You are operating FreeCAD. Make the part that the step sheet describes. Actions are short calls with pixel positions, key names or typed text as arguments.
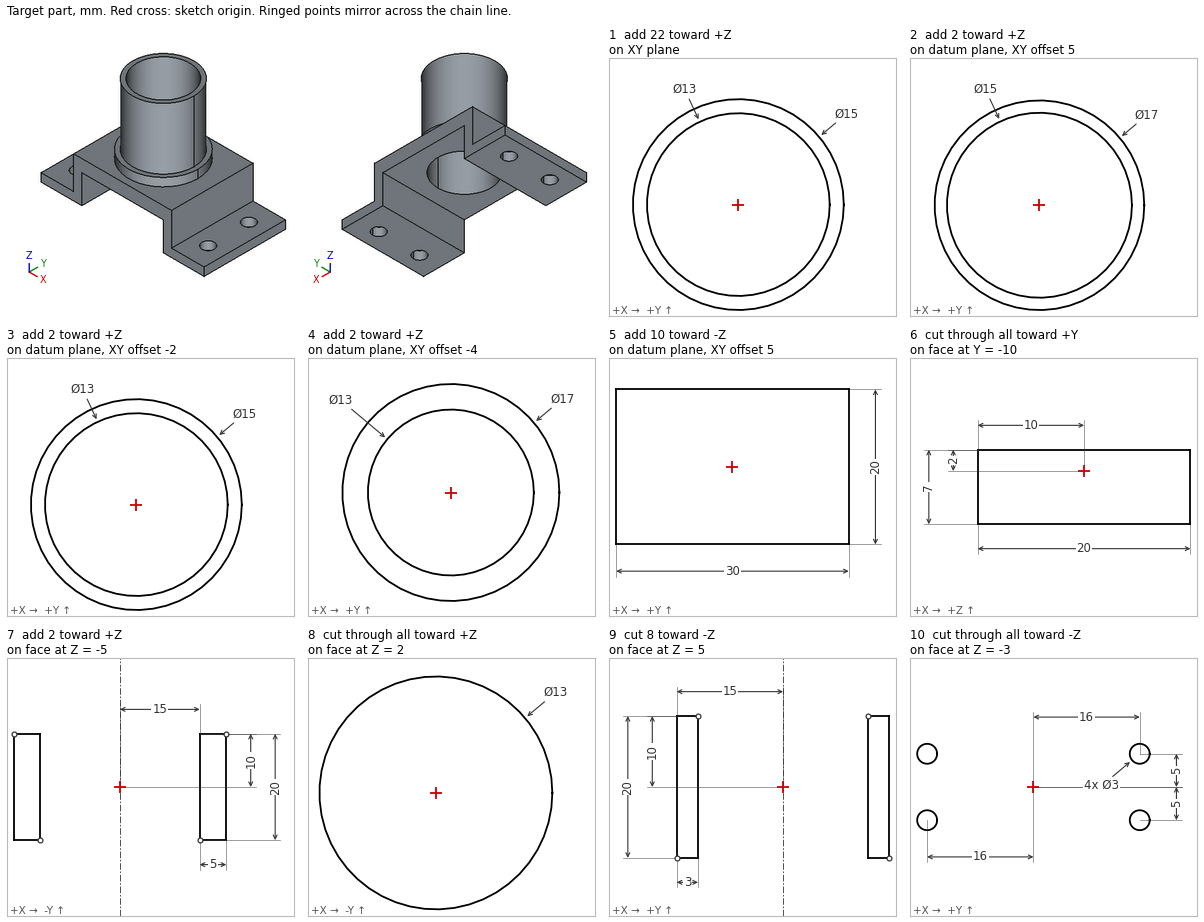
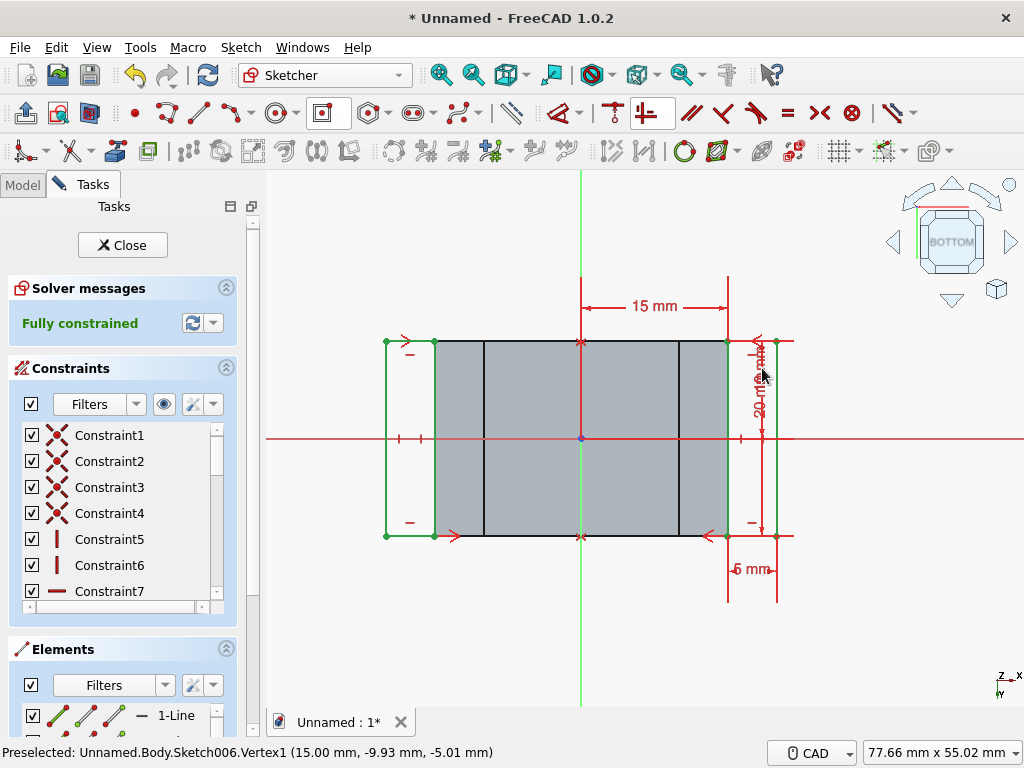
click(123, 245)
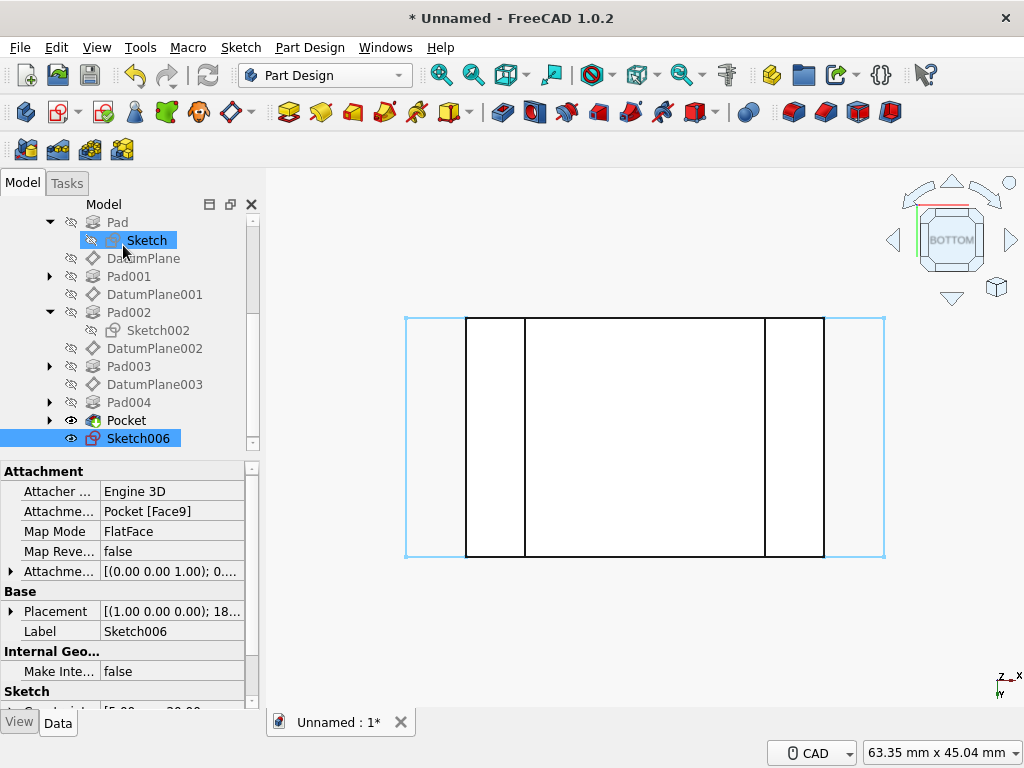
click(290, 112)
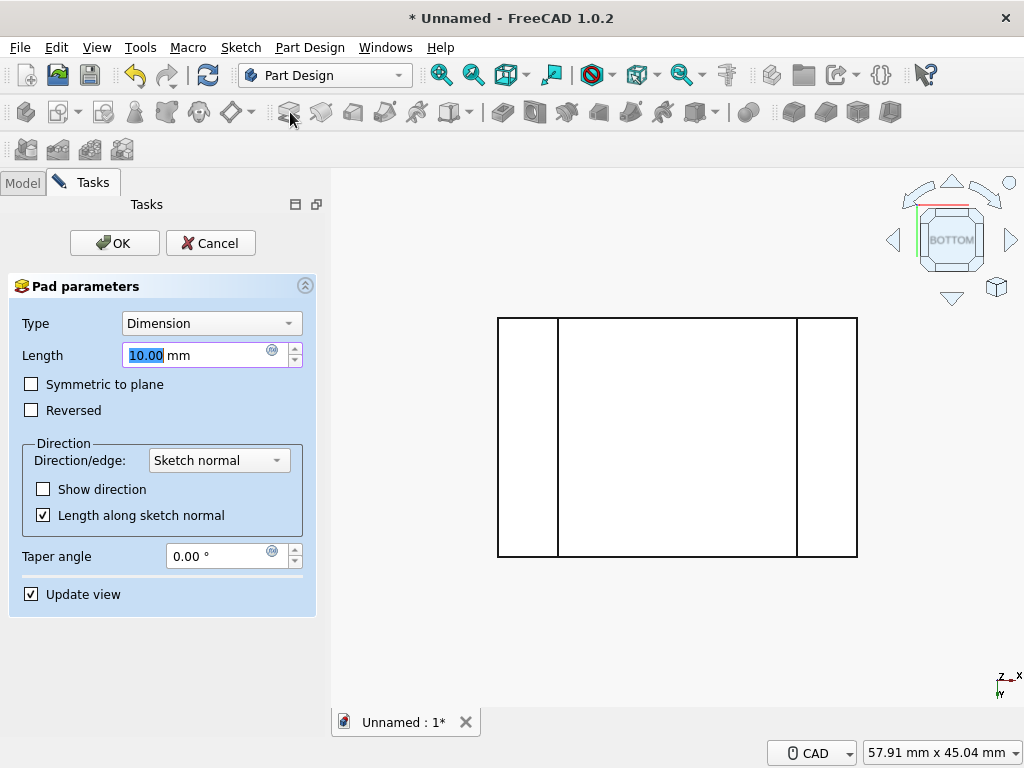
text(2)
key(Tab)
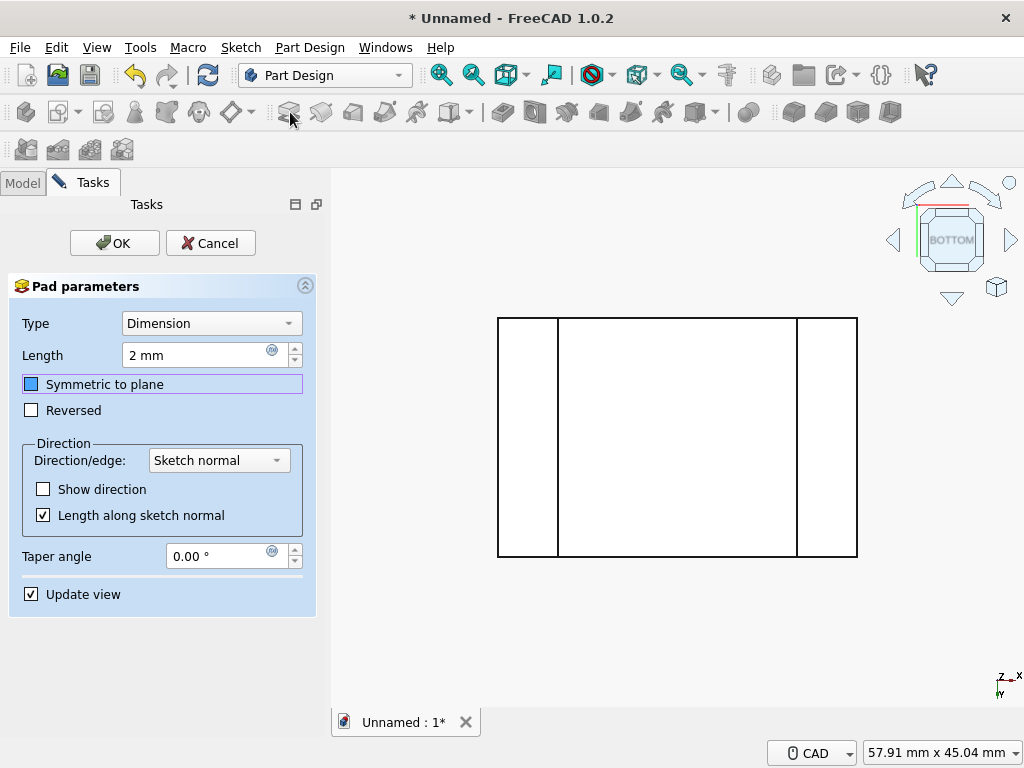
click(30, 410)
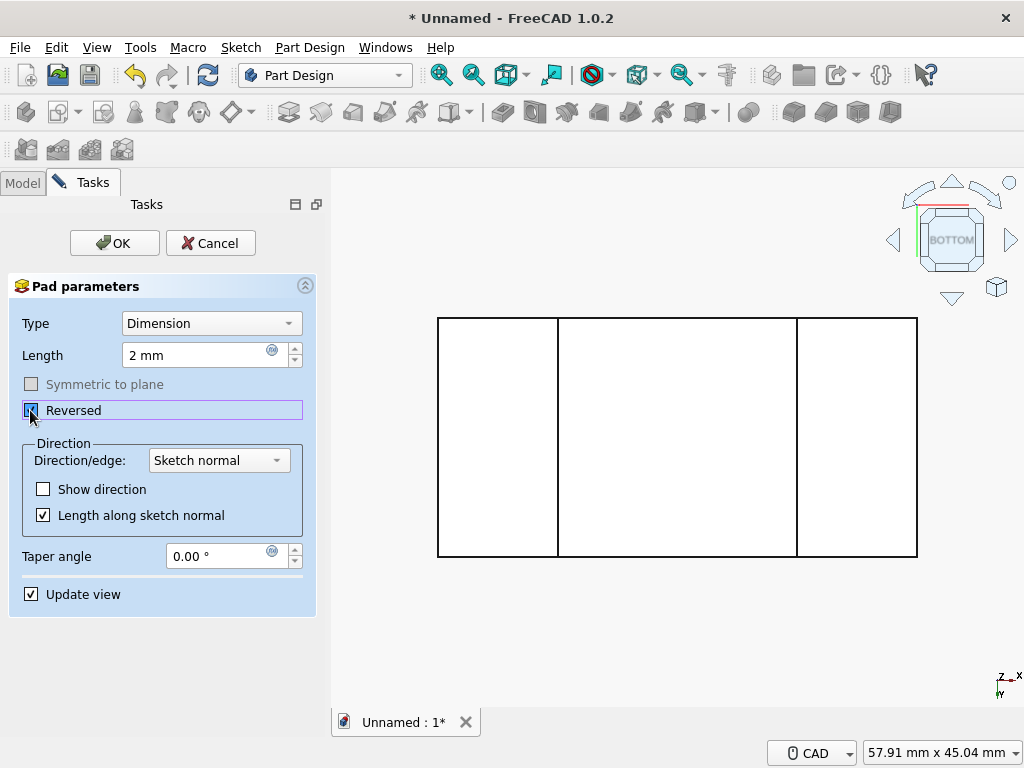
click(115, 243)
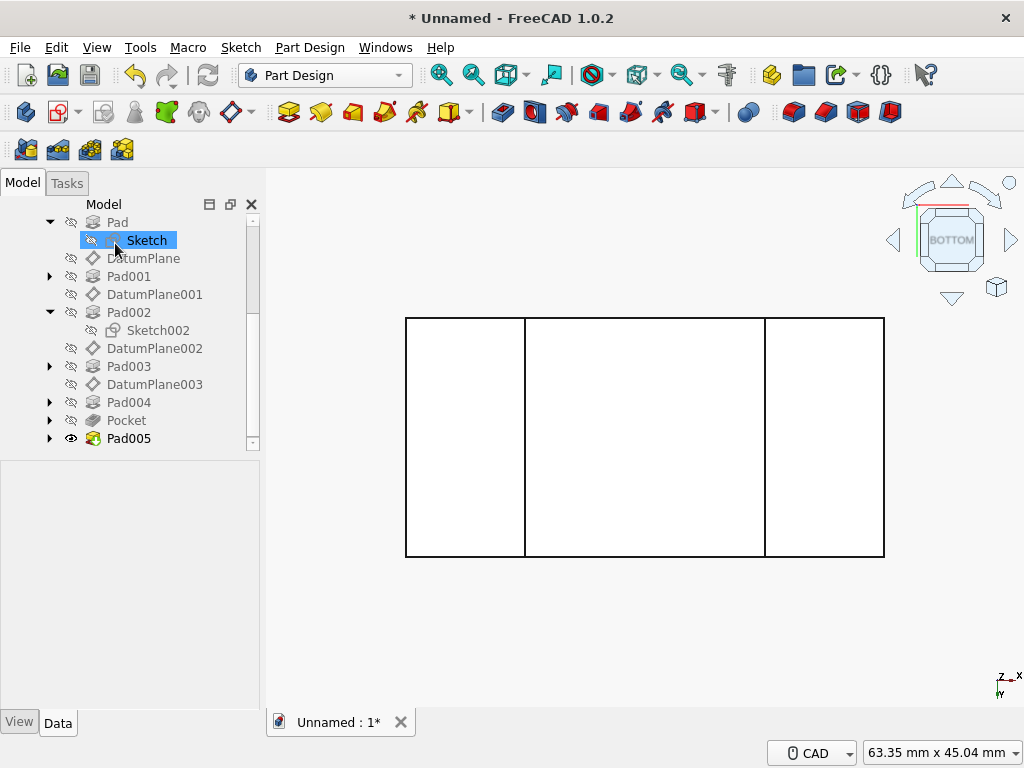
click(645, 437)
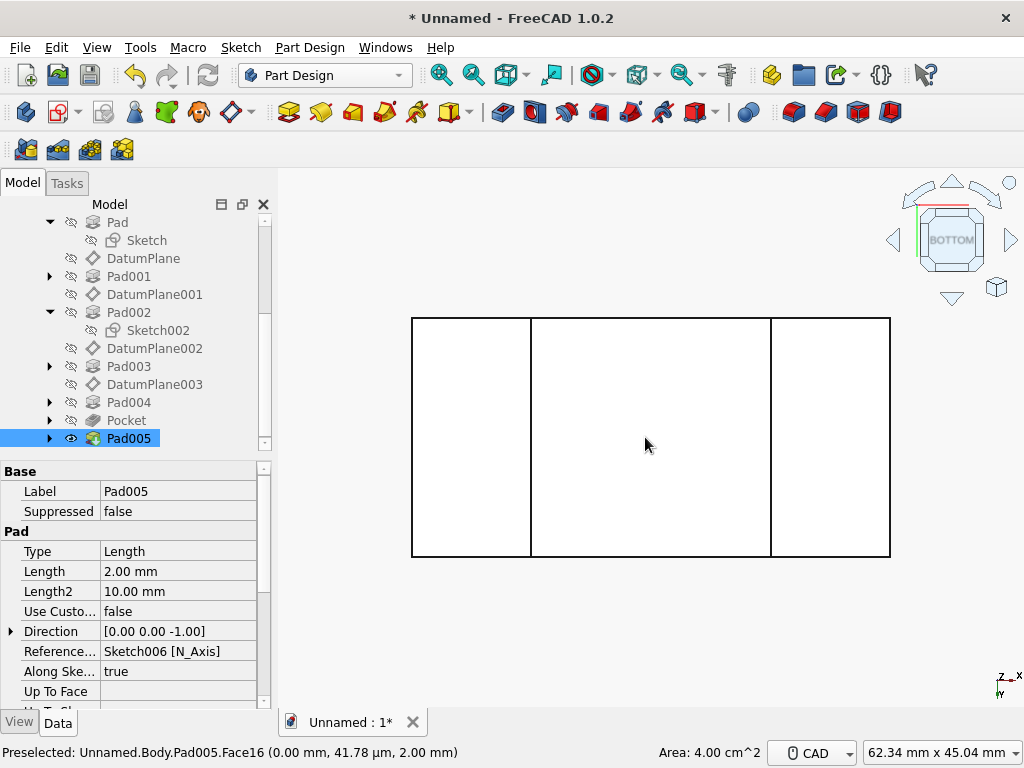
click(58, 112)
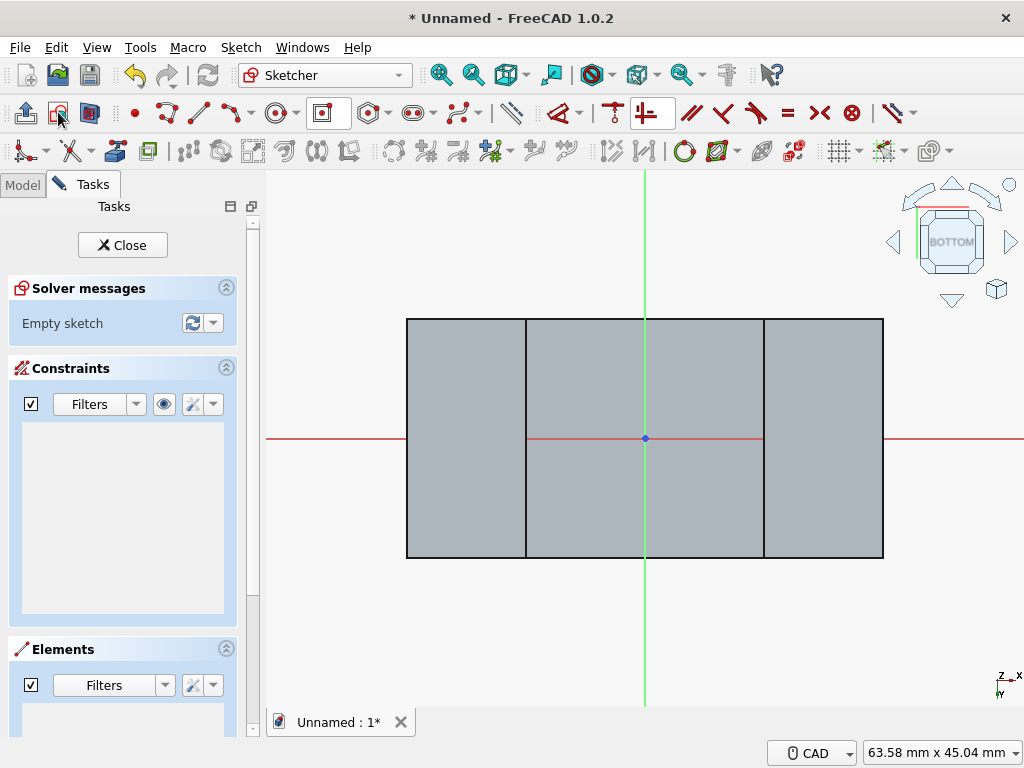
click(90, 114)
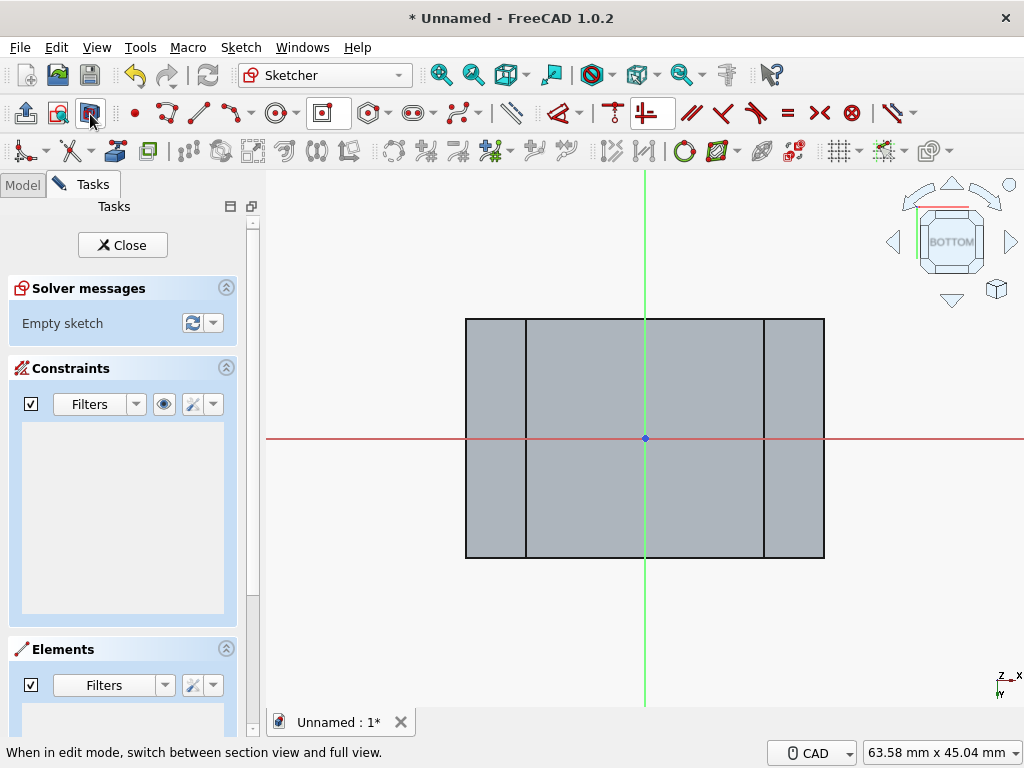
scroll(701, 439, up, 4)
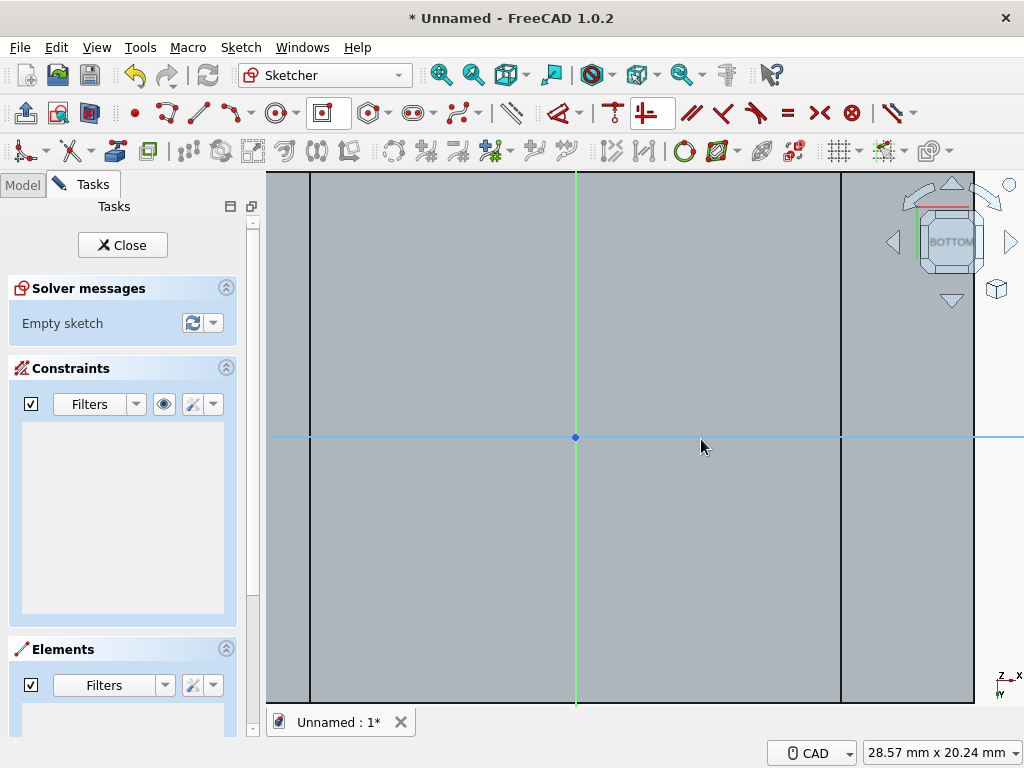
click(276, 114)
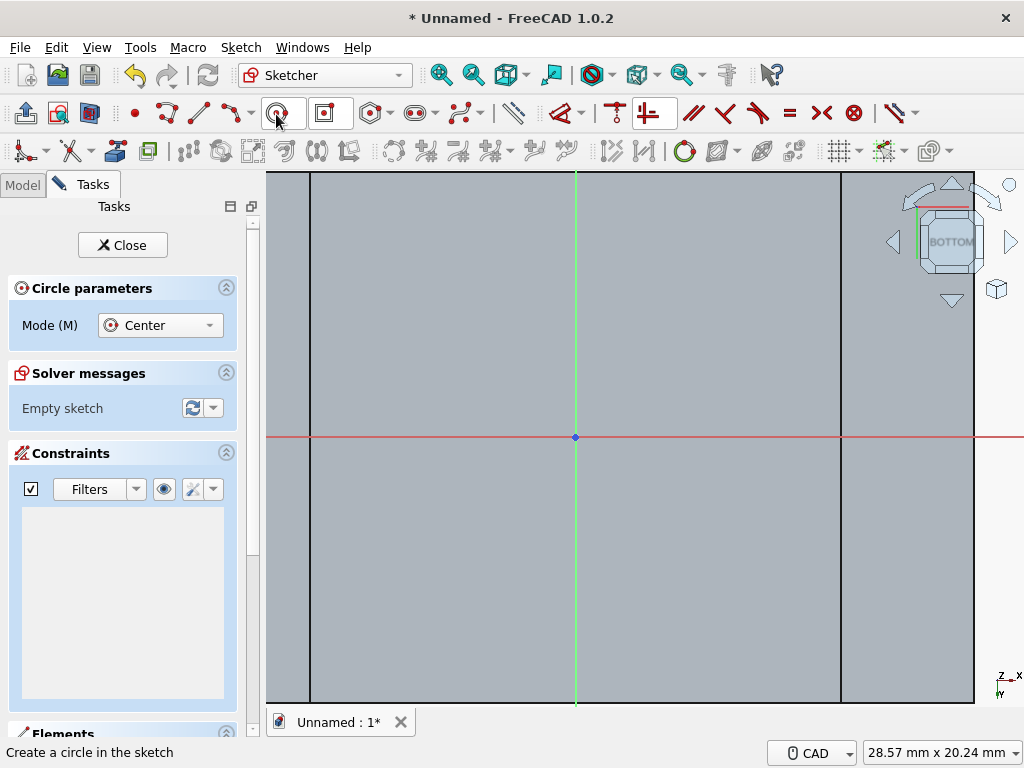
click(576, 437)
click(698, 315)
key(Escape)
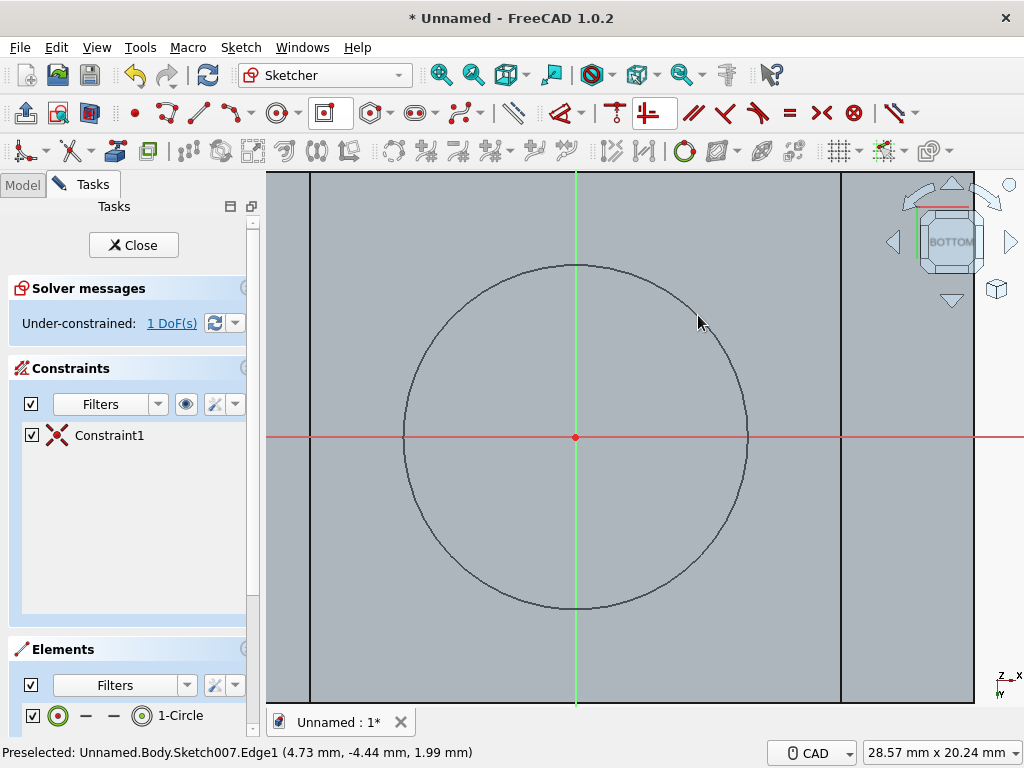
click(560, 114)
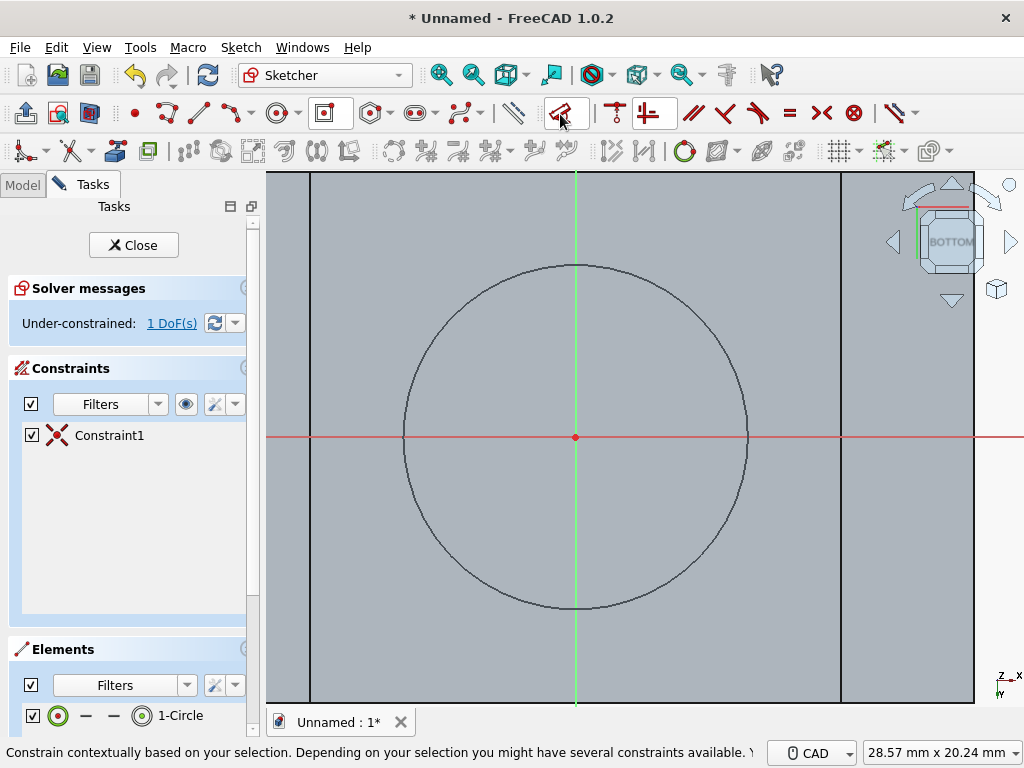
click(697, 315)
click(720, 292)